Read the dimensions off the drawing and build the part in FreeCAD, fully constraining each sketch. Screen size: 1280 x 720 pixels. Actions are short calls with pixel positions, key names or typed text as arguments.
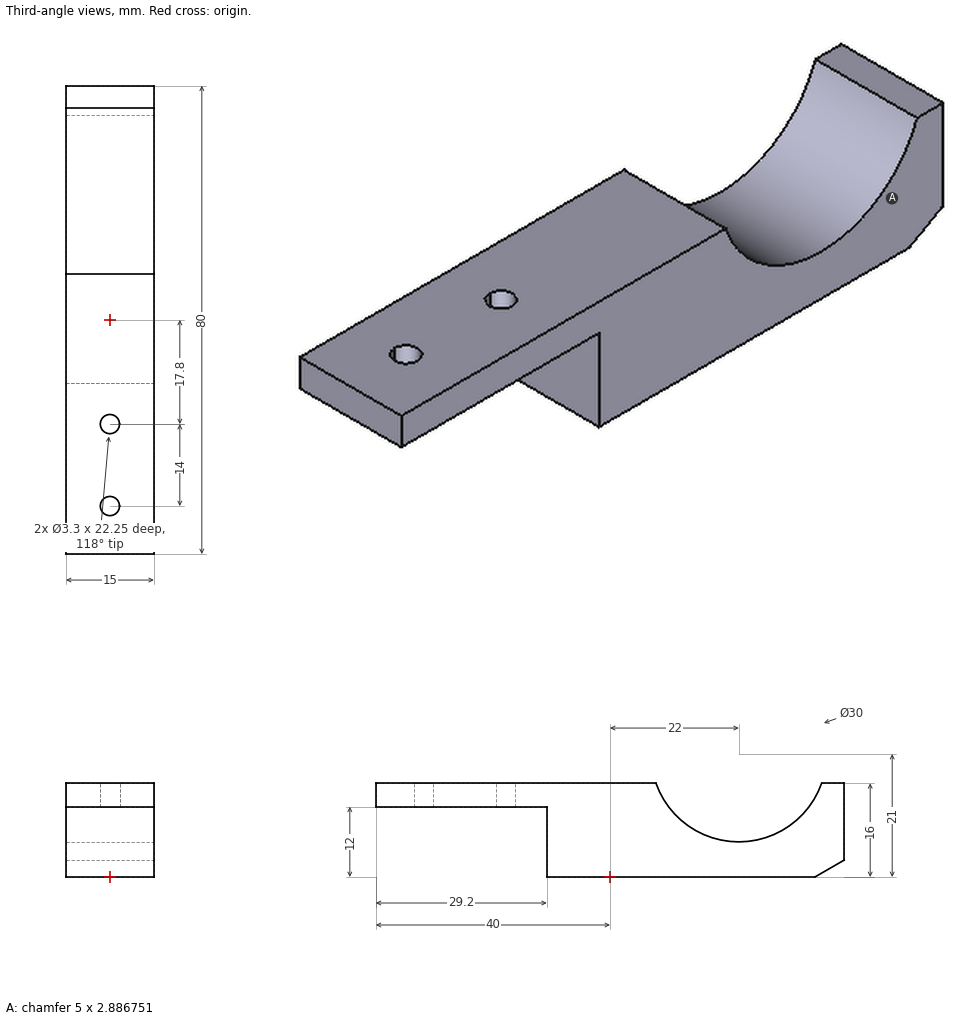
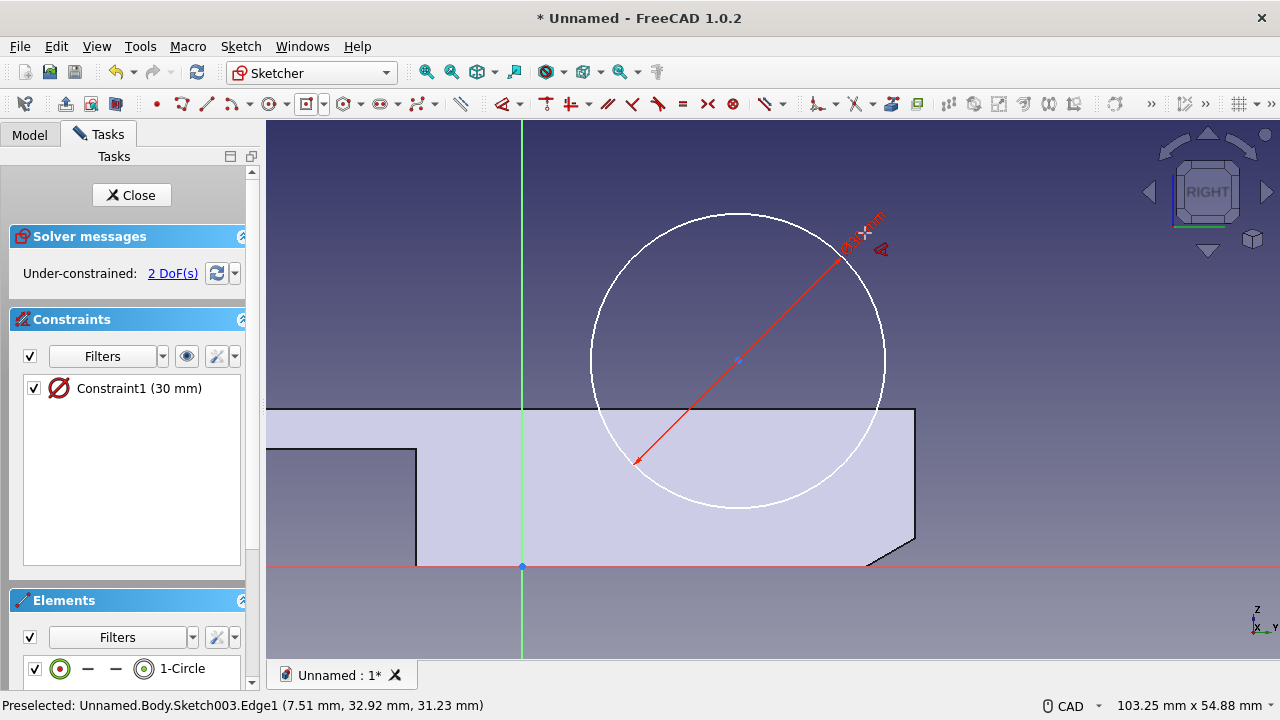
click(738, 361)
click(630, 601)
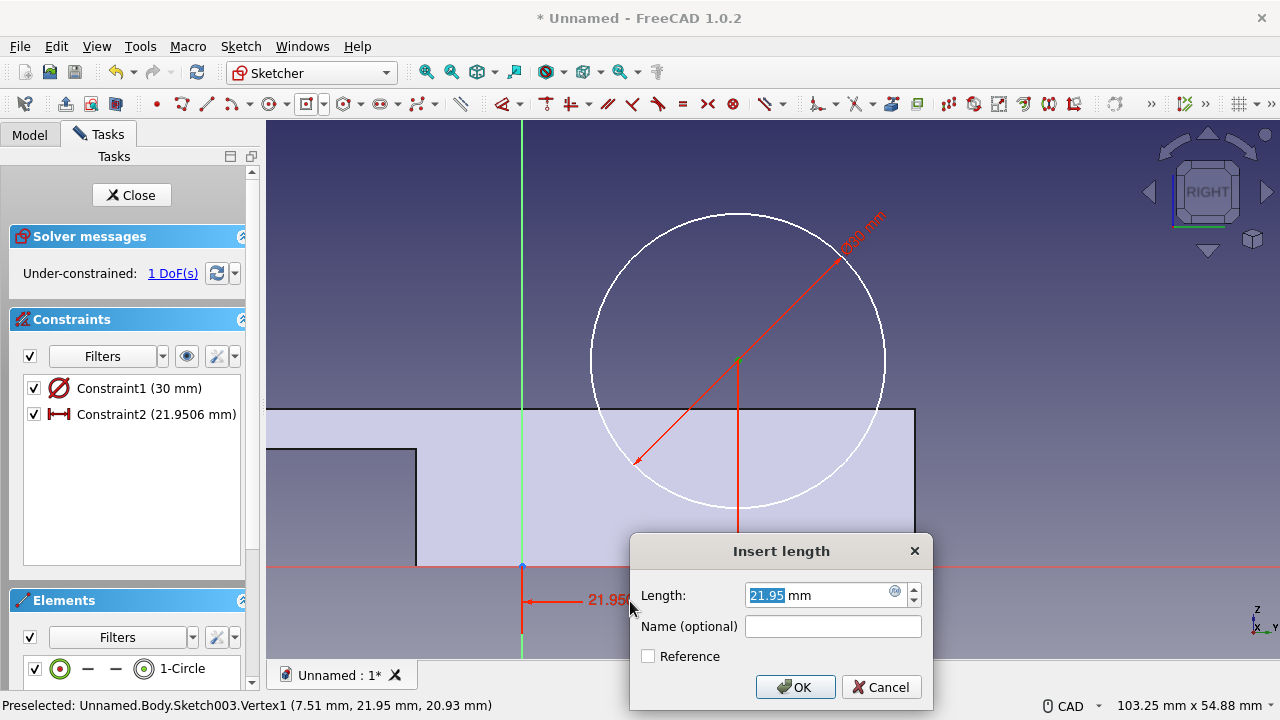
text(22)
key(Return)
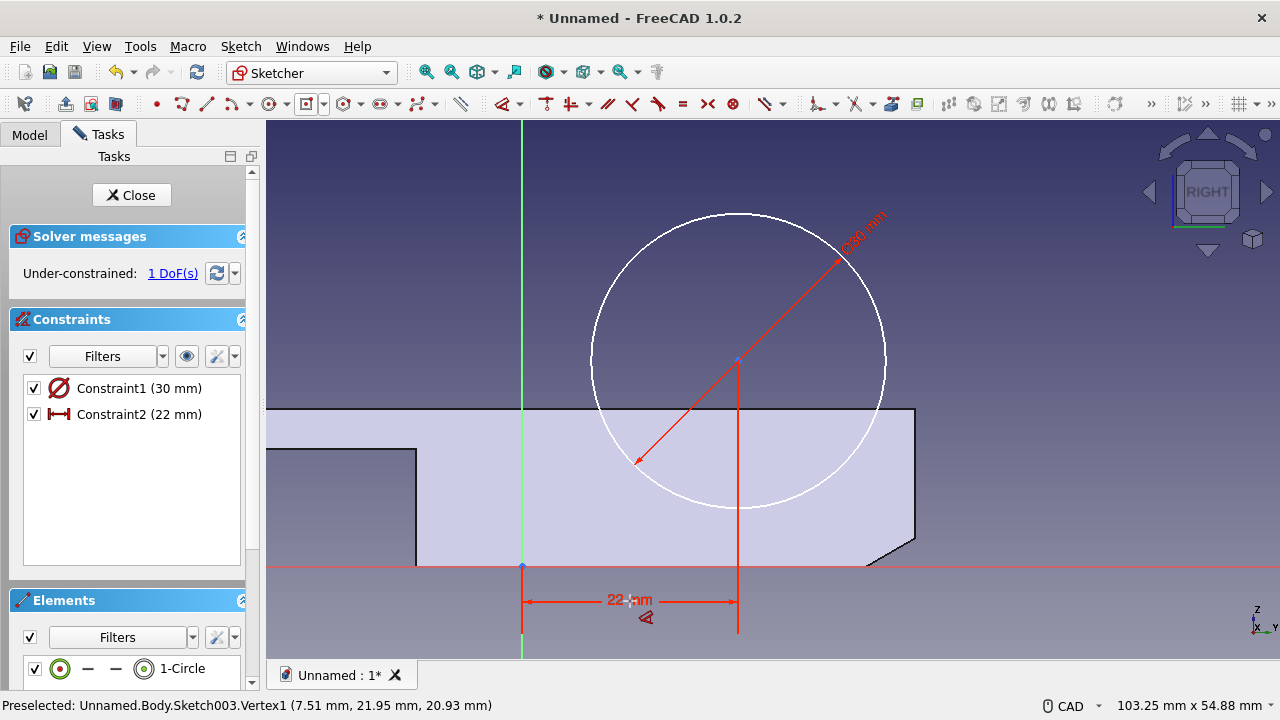
click(738, 361)
click(488, 464)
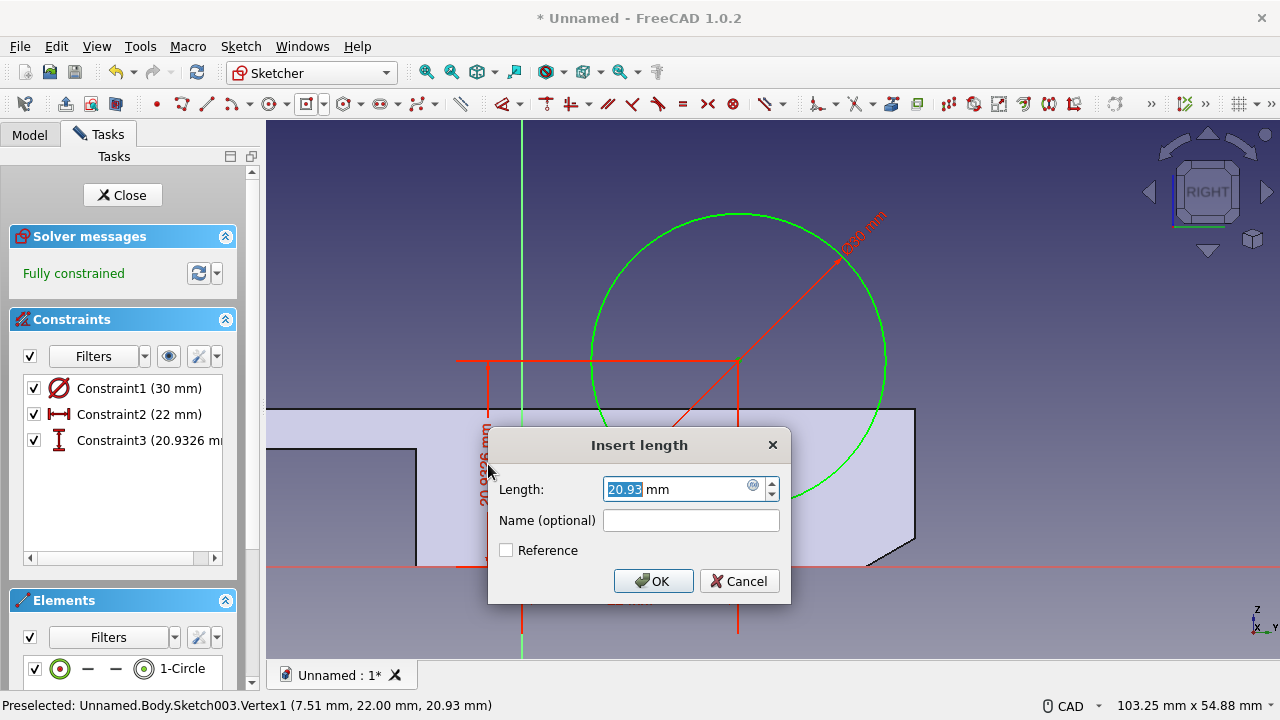
text(21)
key(Return)
key(Escape)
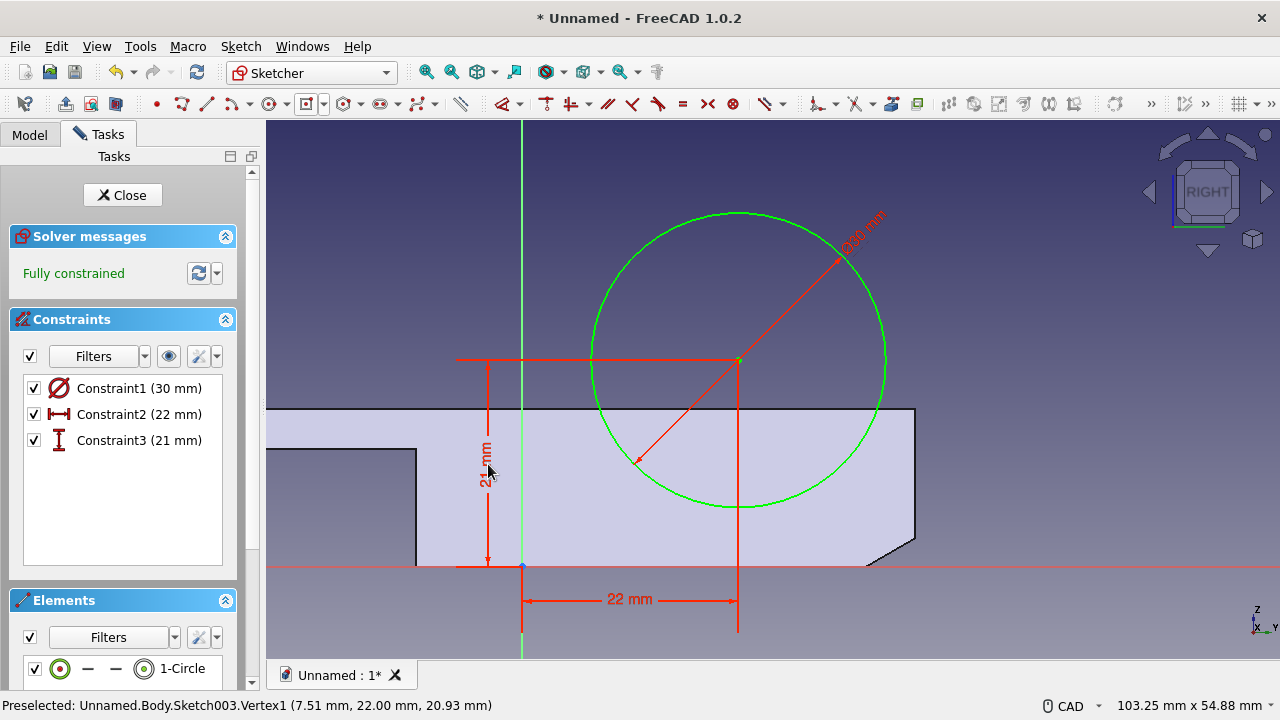
click(123, 195)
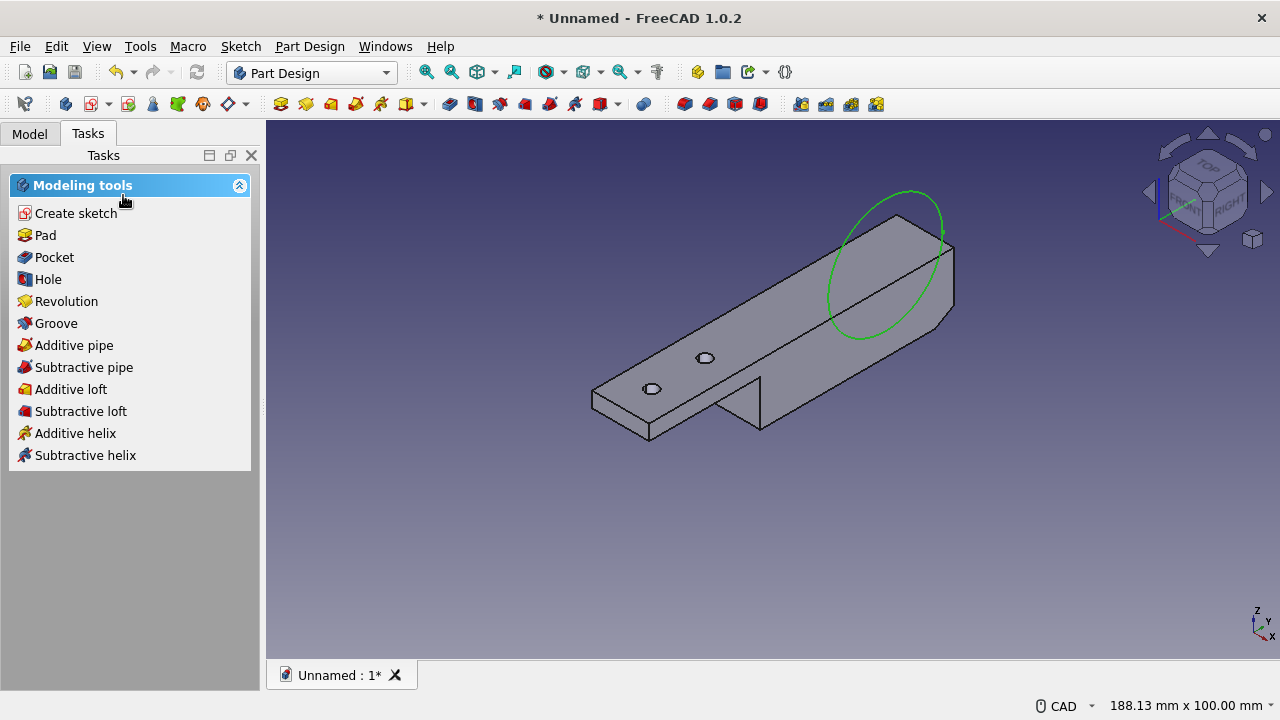
click(450, 104)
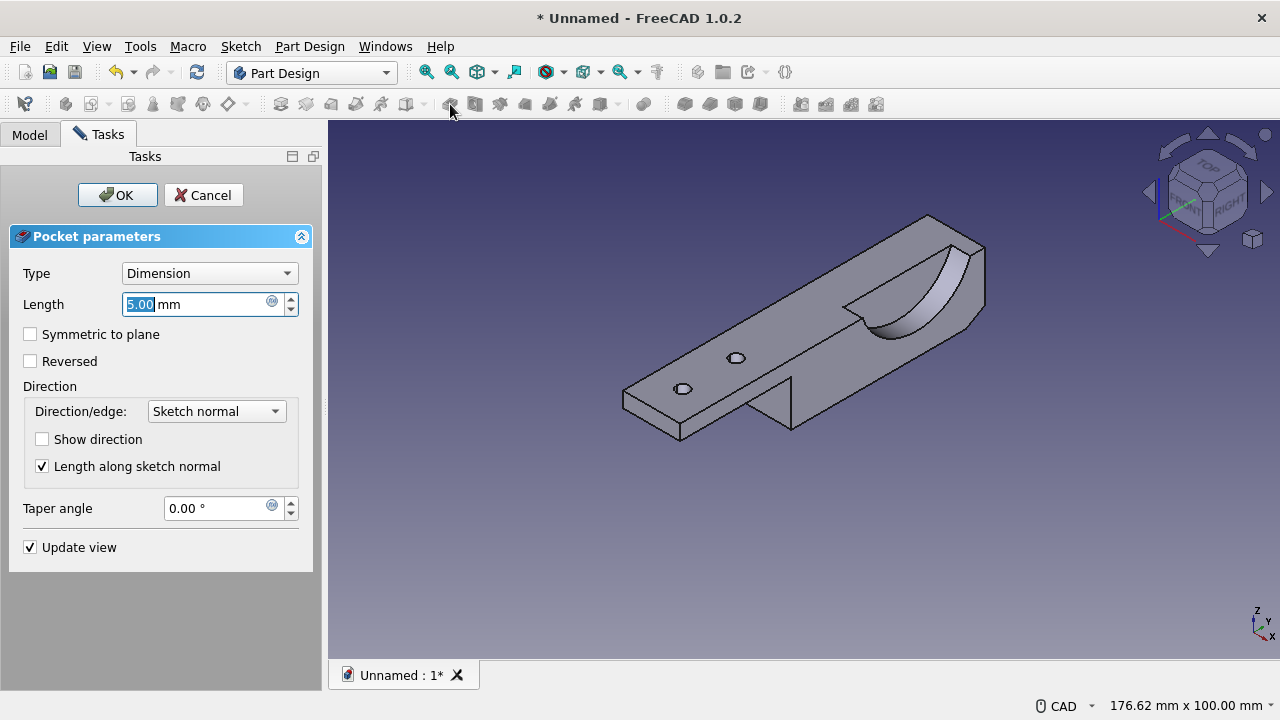
click(210, 274)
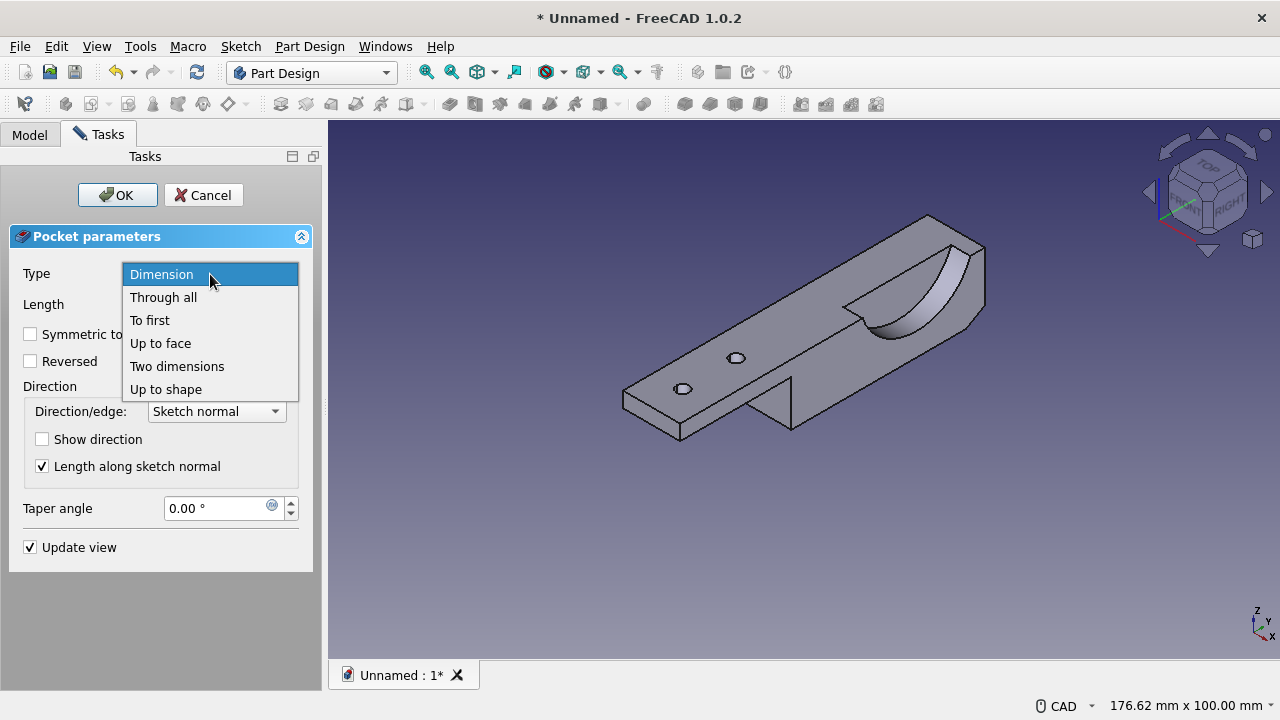
click(208, 298)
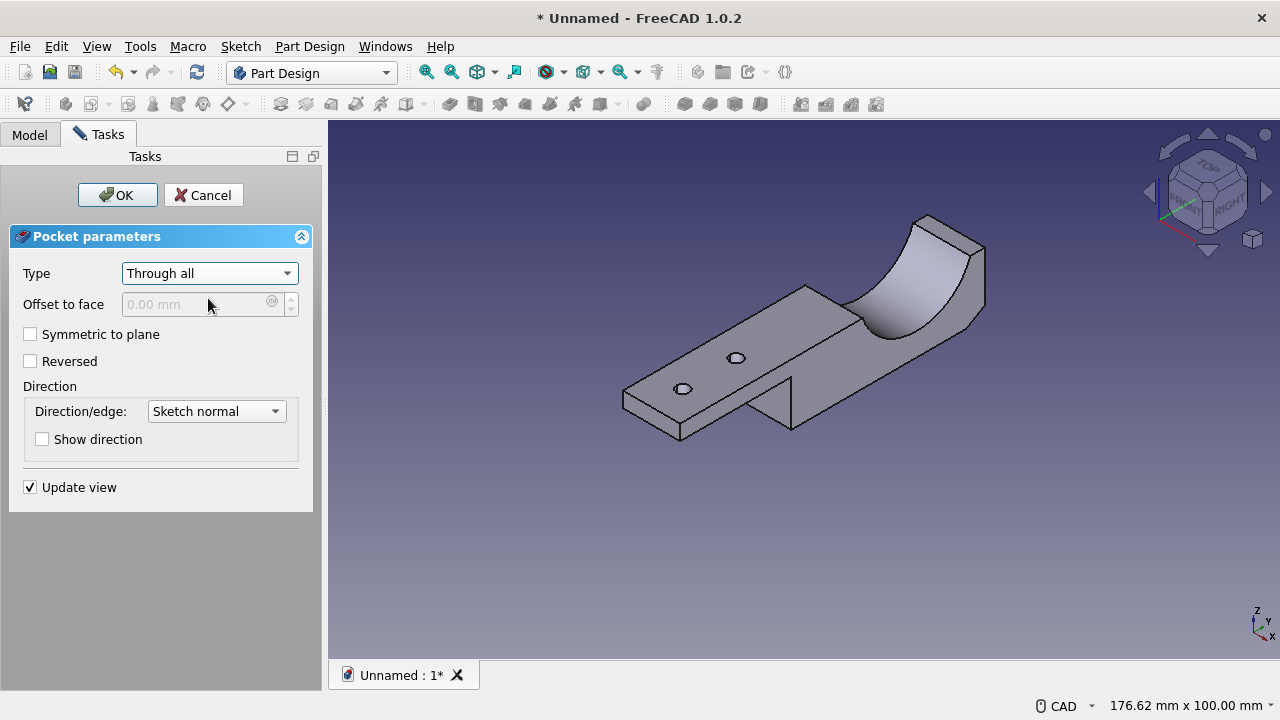
click(118, 195)